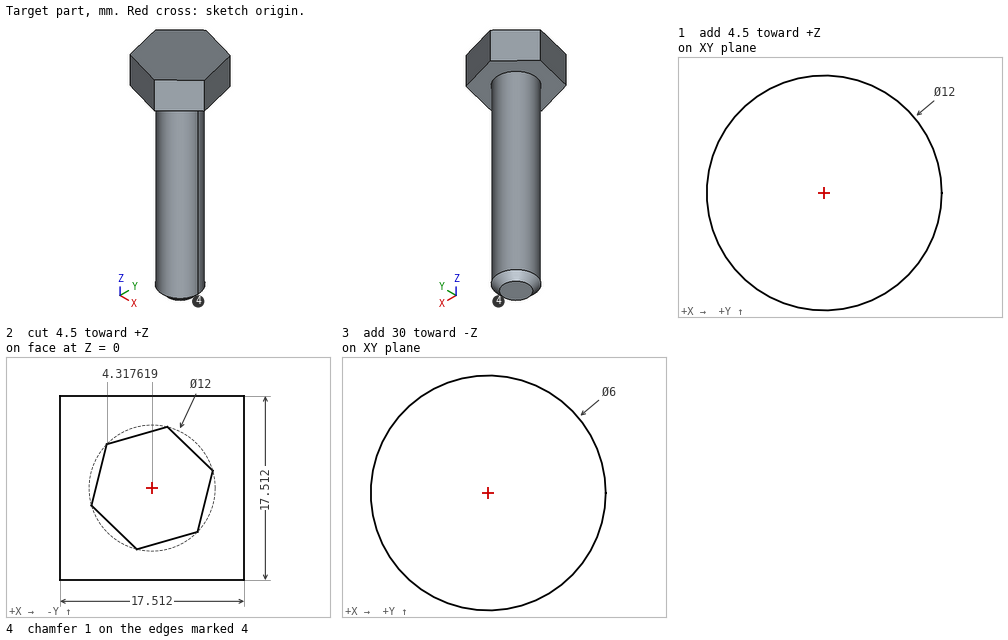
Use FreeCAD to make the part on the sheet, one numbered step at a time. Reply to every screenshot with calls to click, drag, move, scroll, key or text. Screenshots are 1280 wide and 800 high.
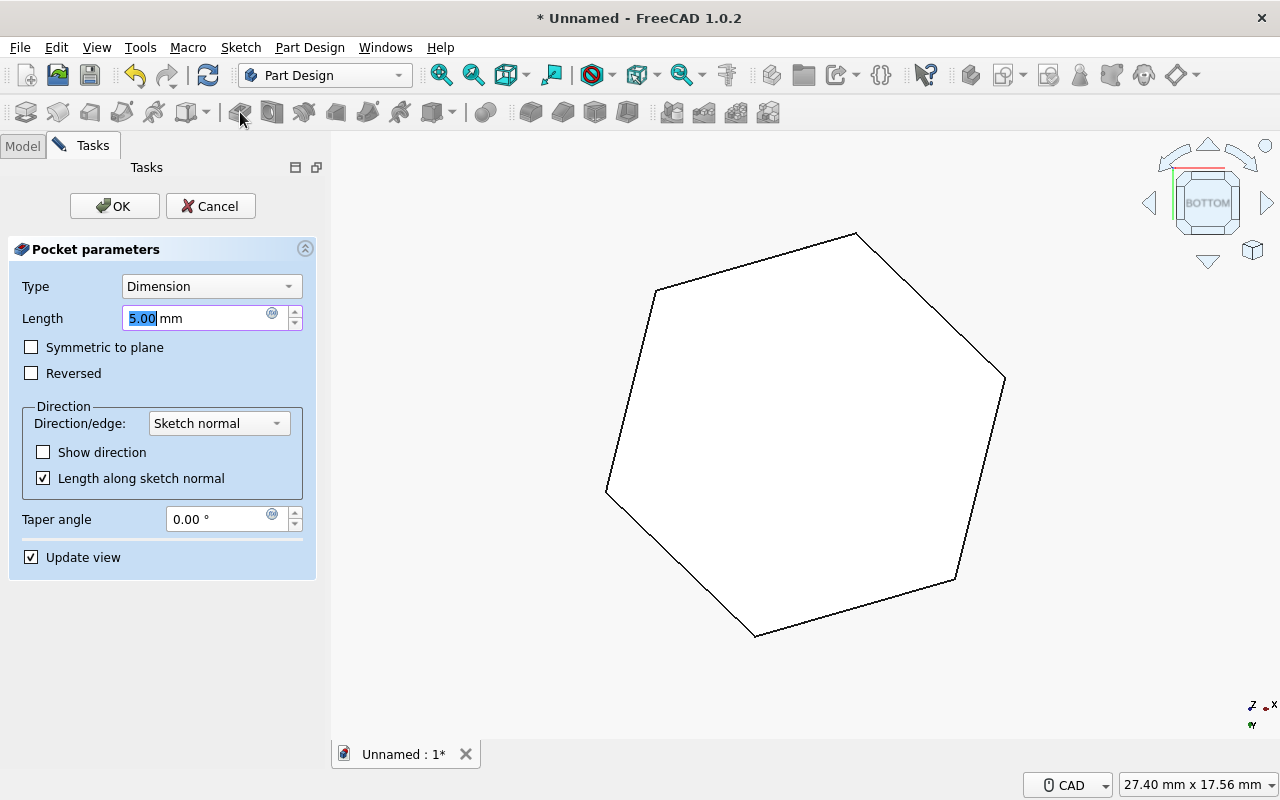
text(4.5)
key(Tab)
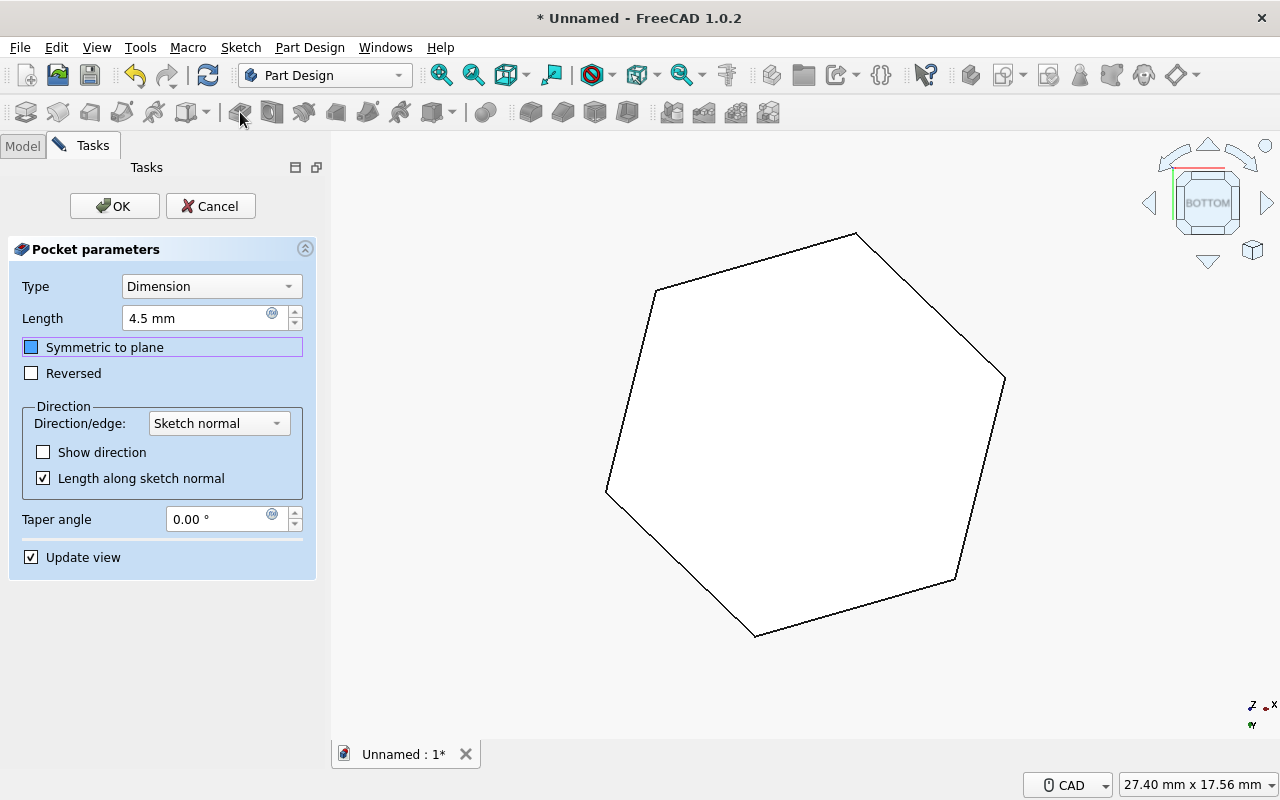
click(115, 206)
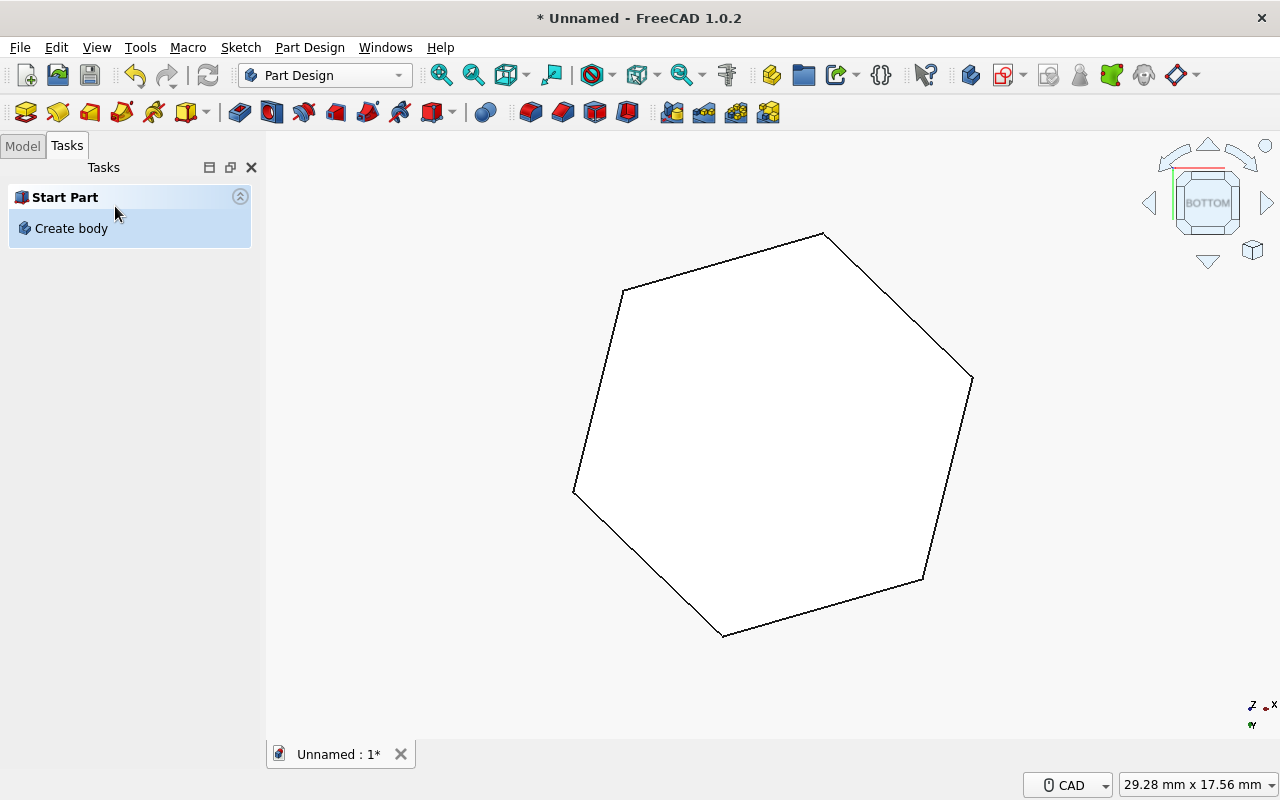
click(1004, 76)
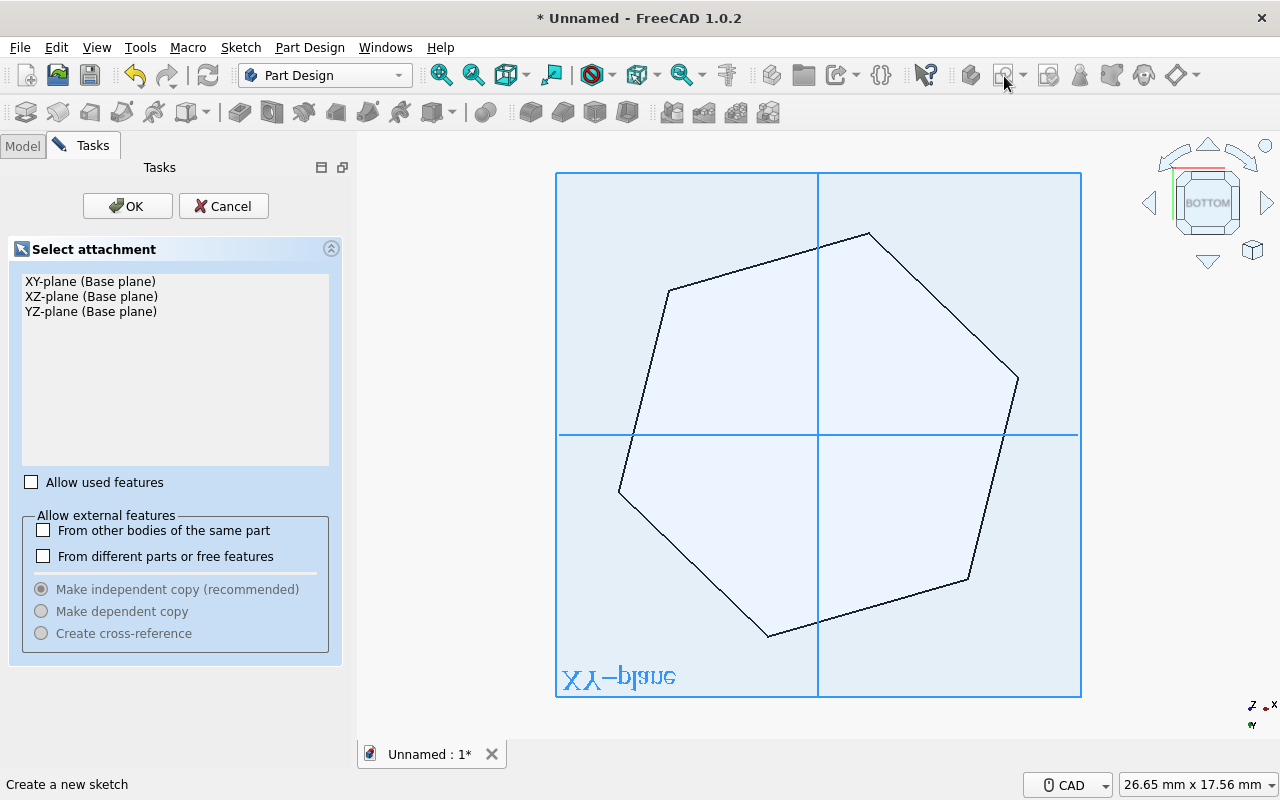
click(82, 282)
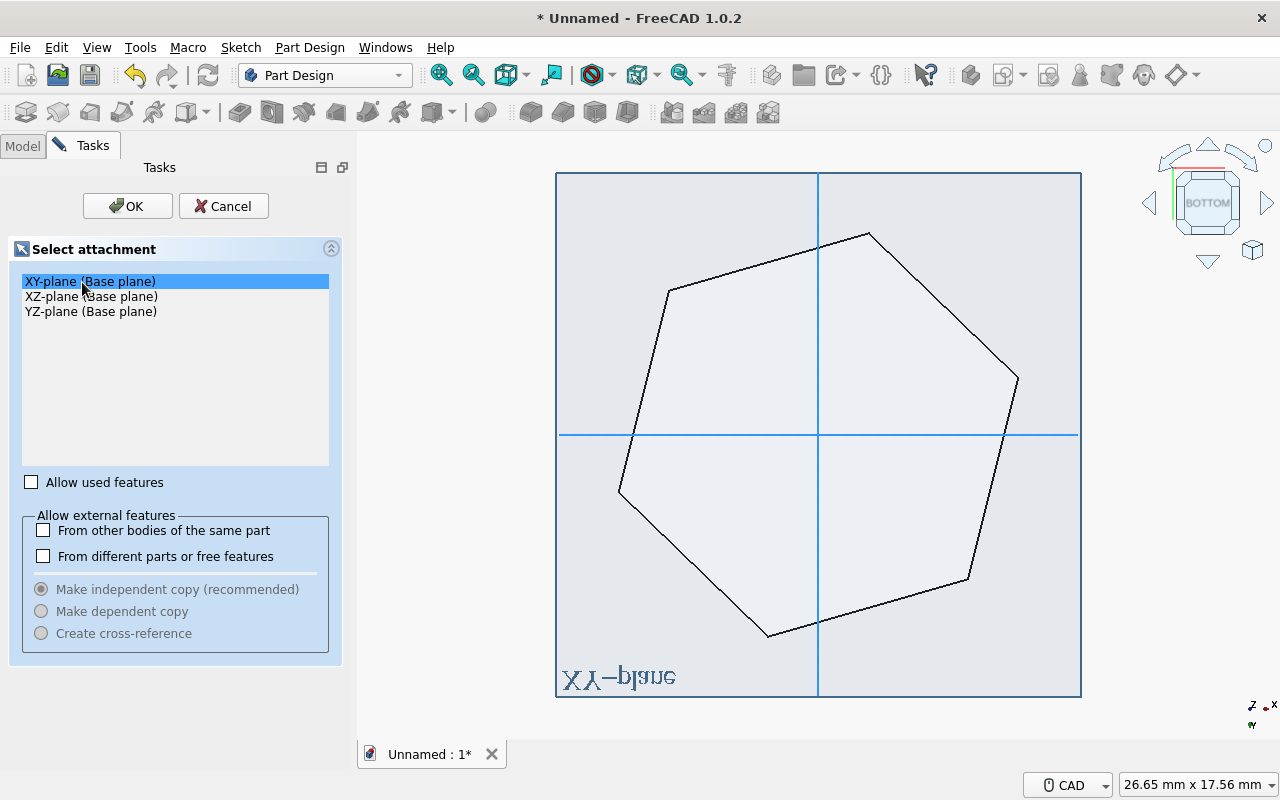
click(128, 206)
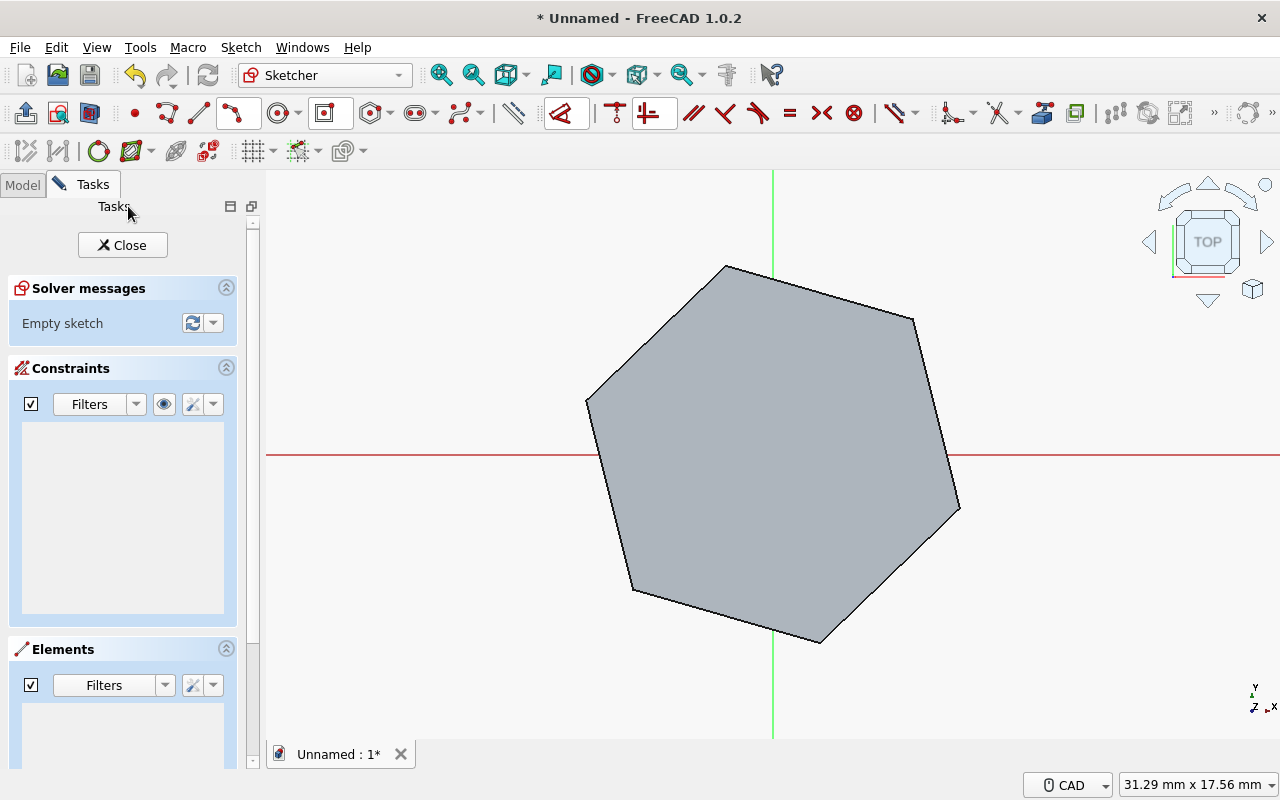
click(90, 114)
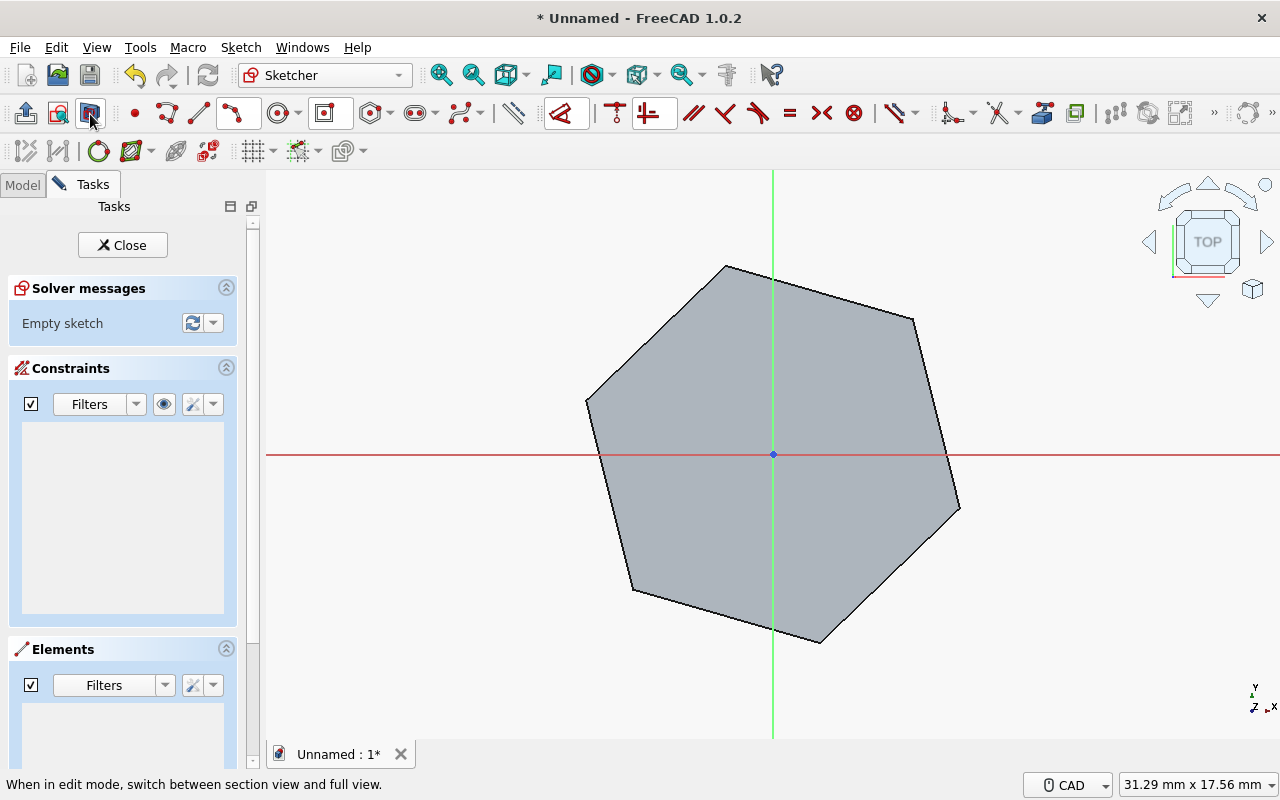
scroll(856, 454, up, 3)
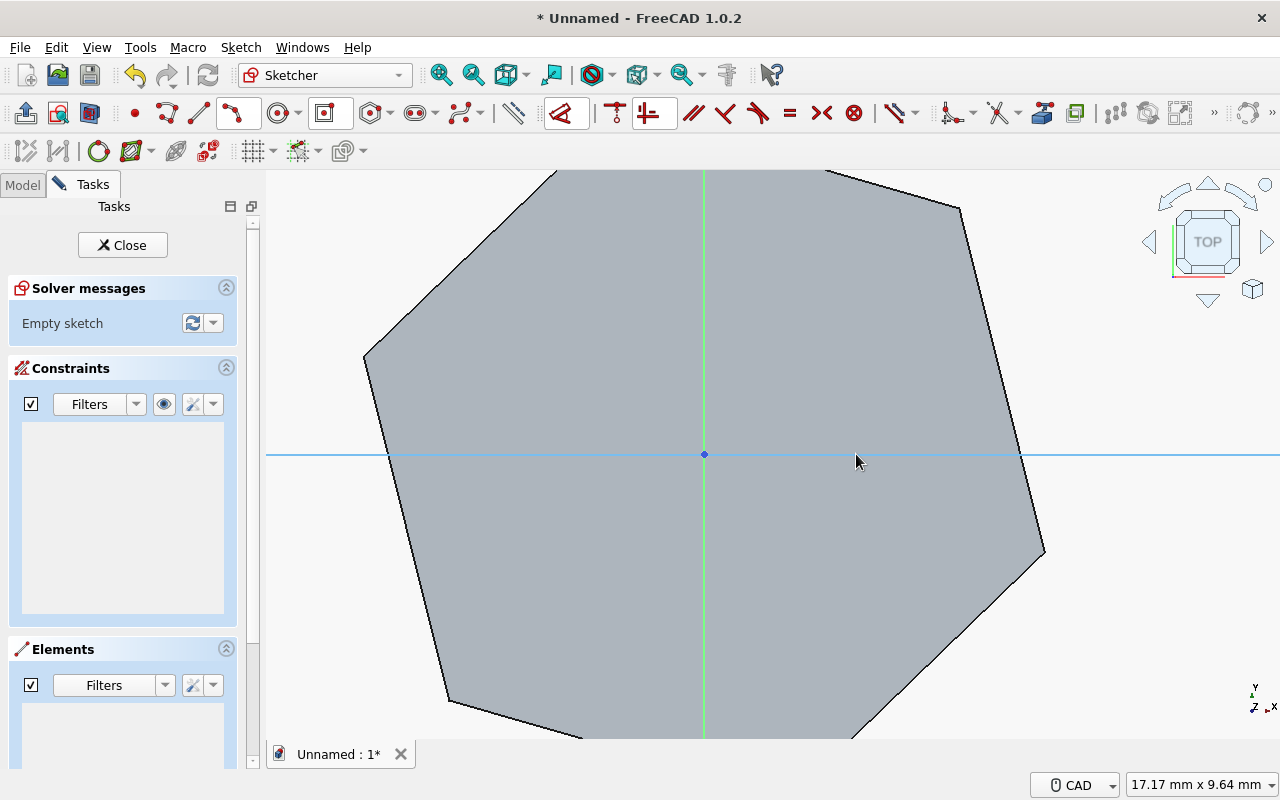
click(278, 114)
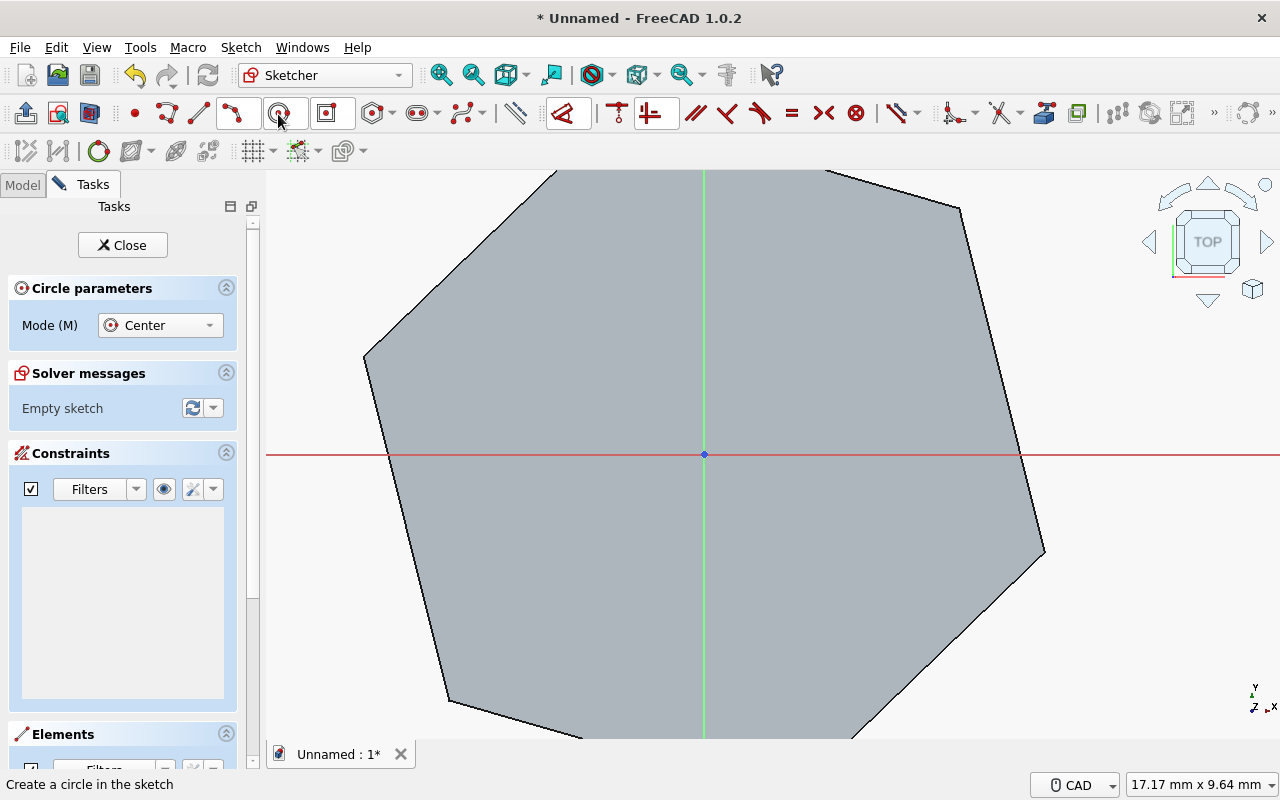
click(704, 454)
click(830, 329)
key(Escape)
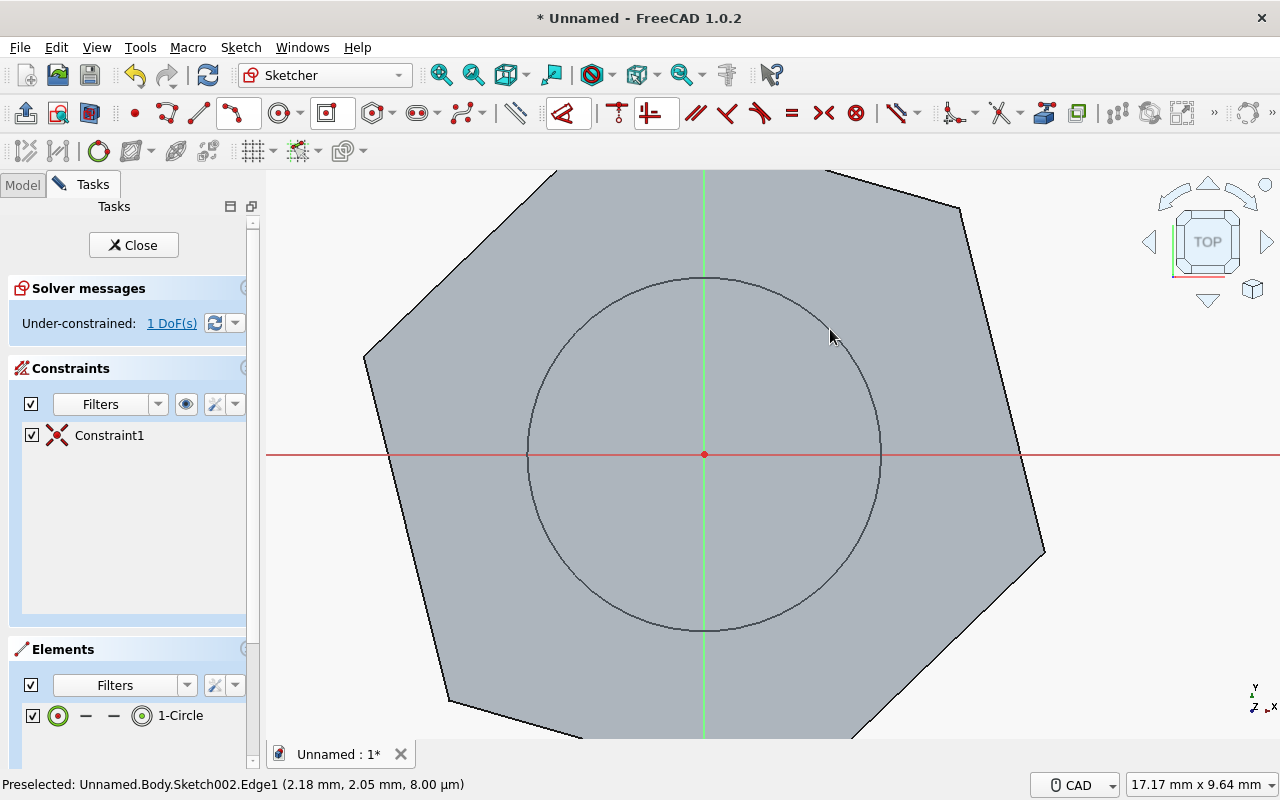
click(829, 329)